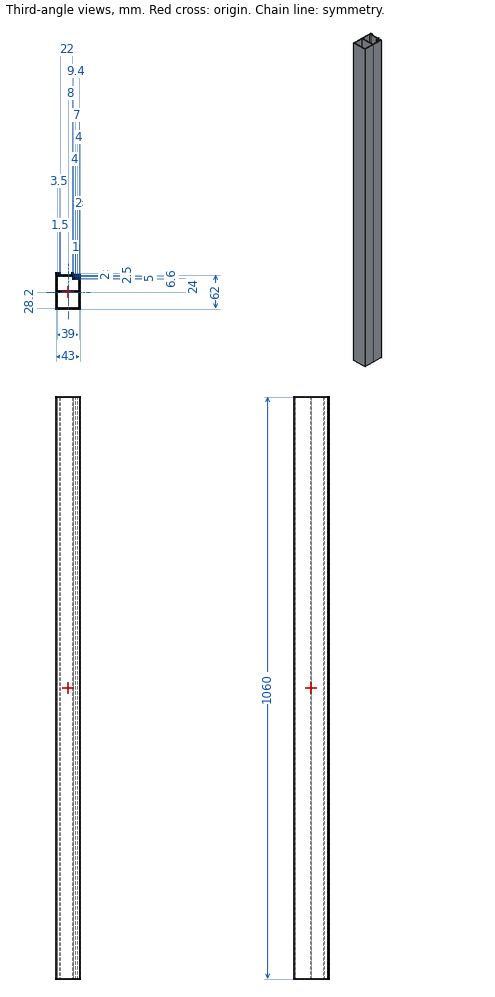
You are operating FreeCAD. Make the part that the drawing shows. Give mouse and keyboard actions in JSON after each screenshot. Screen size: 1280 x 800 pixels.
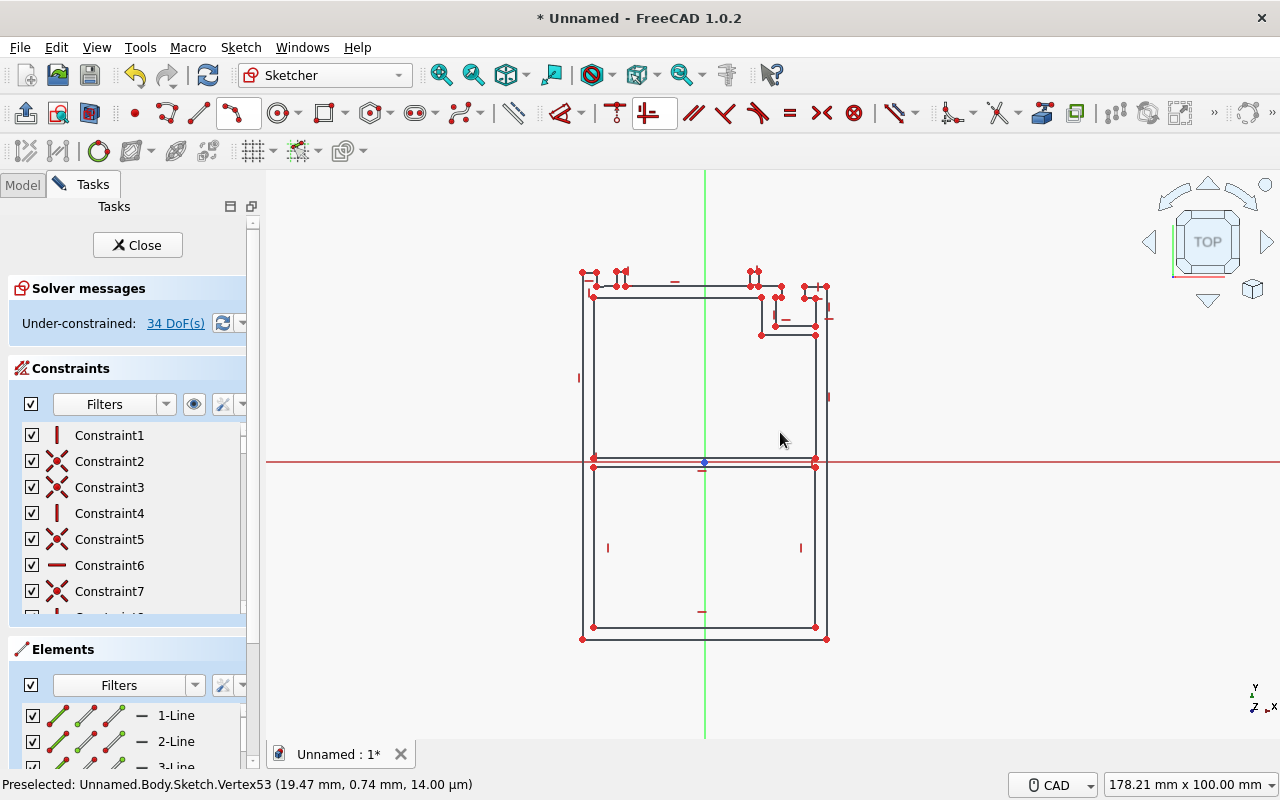
{"action": "scroll", "coordinate": [778, 298], "scroll_direction": "up", "scroll_amount": 9}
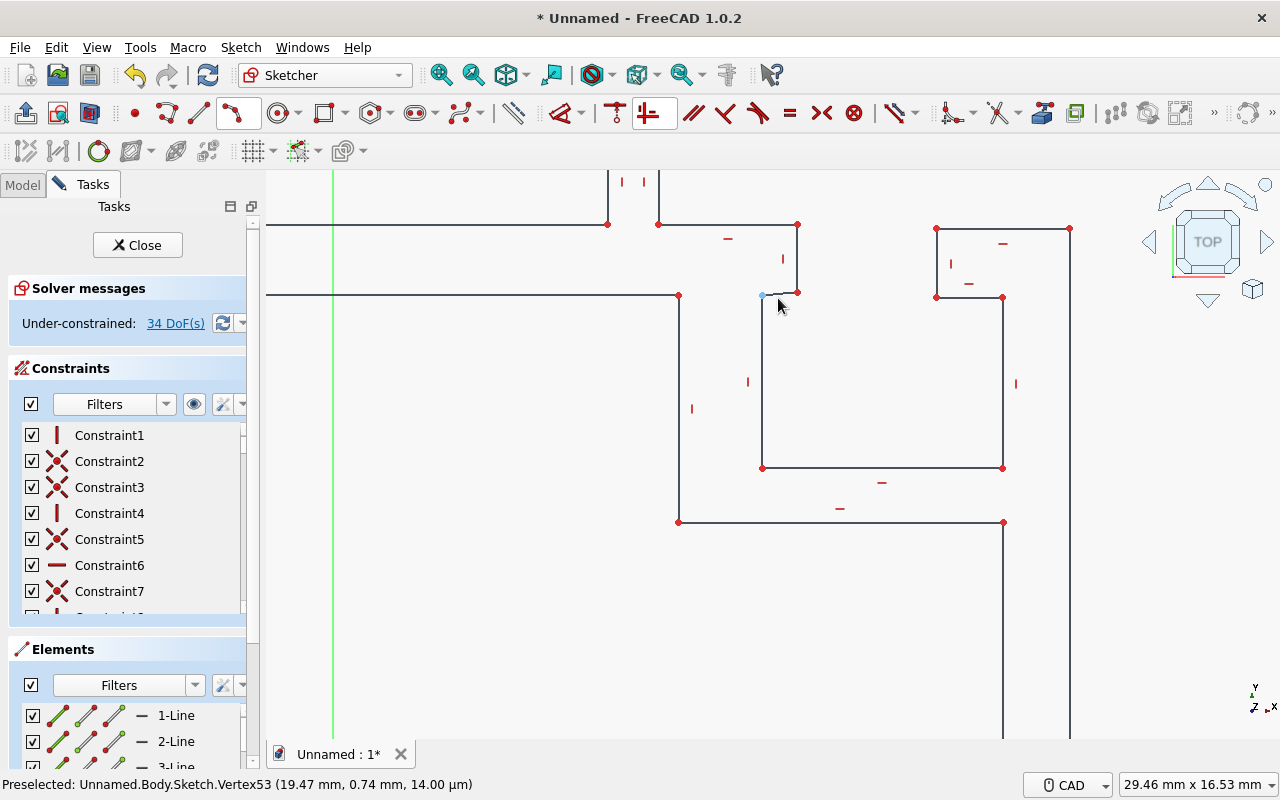
{"action": "left_click", "coordinate": [776, 294]}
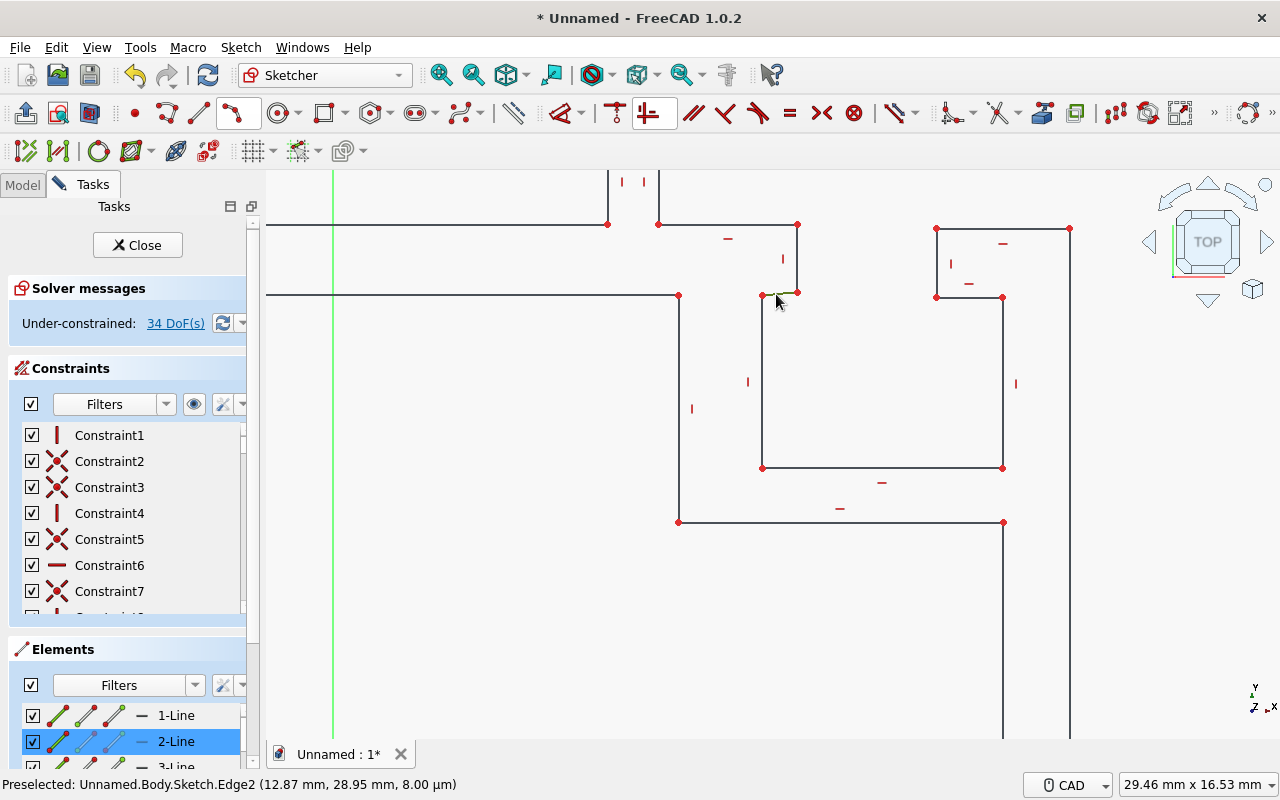
{"action": "left_click", "coordinate": [672, 114]}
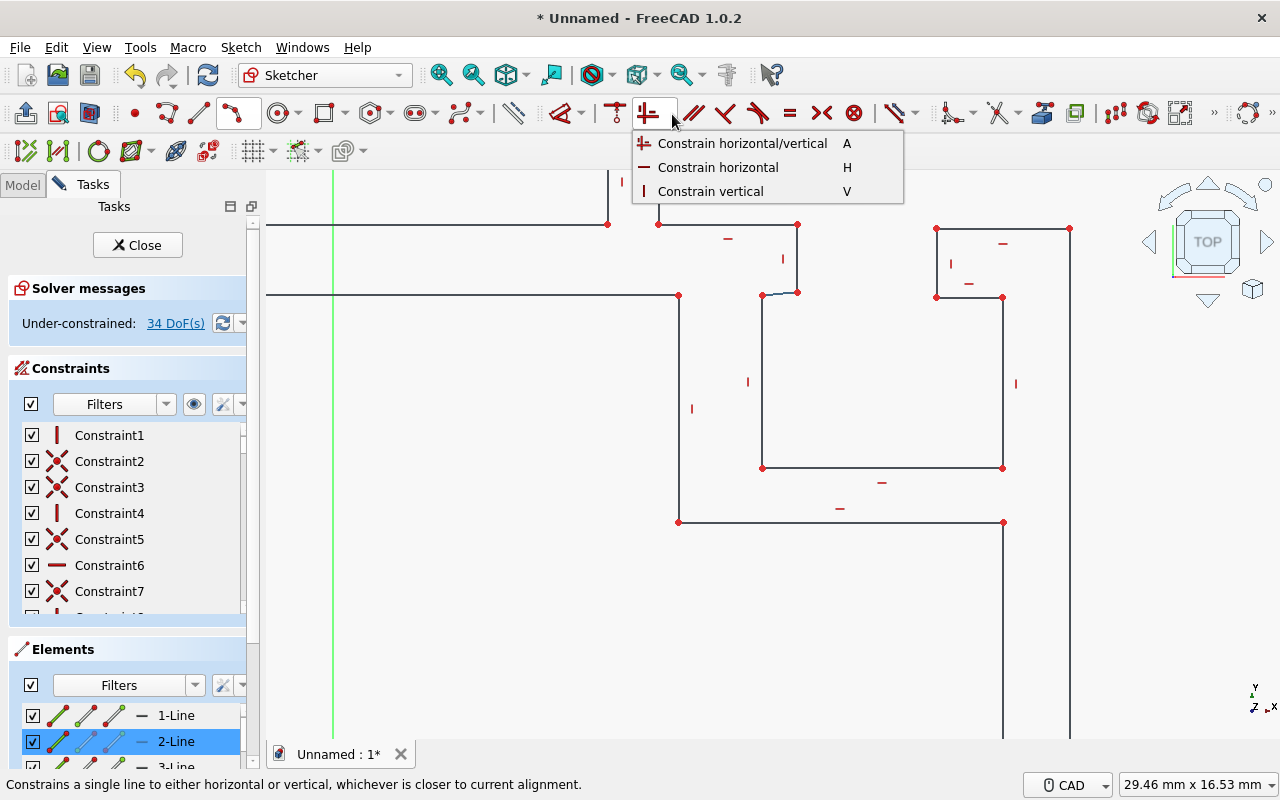
{"action": "left_click", "coordinate": [768, 167]}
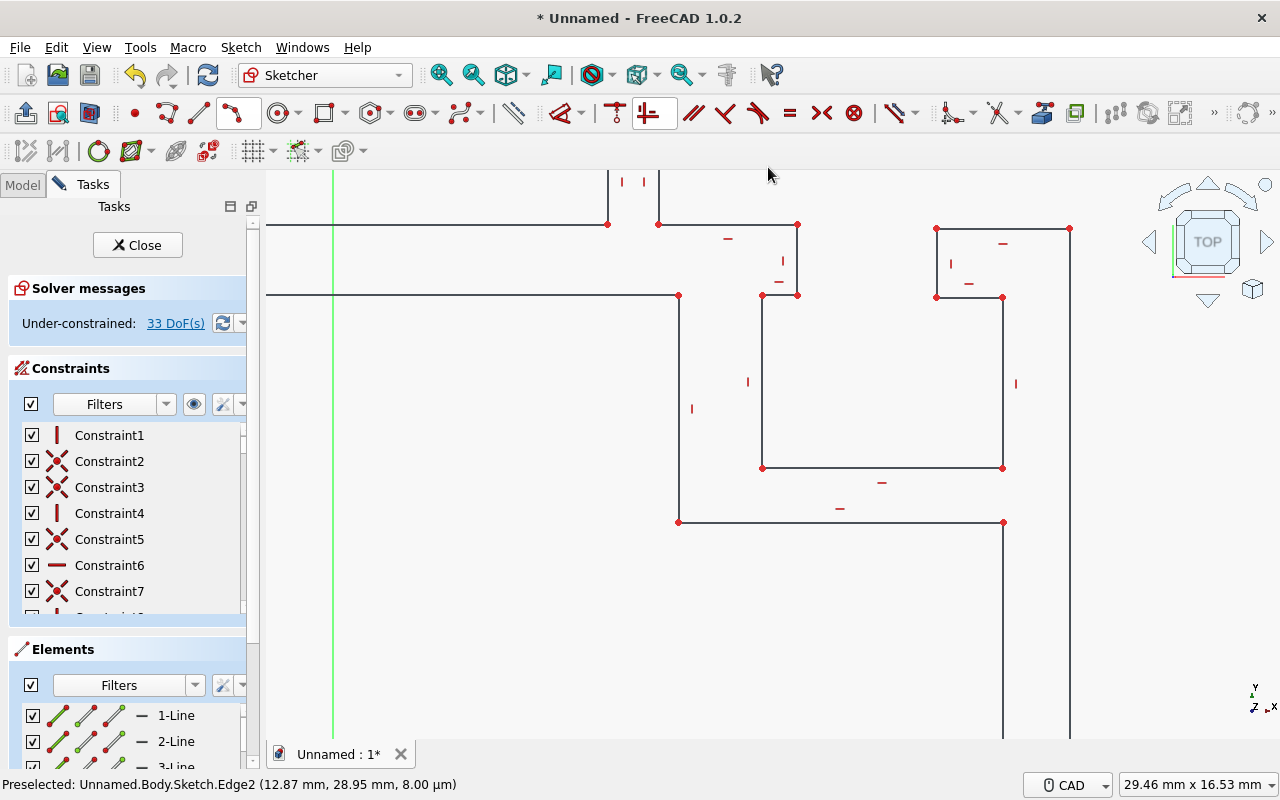
{"action": "scroll", "coordinate": [778, 297], "scroll_direction": "down", "scroll_amount": 9}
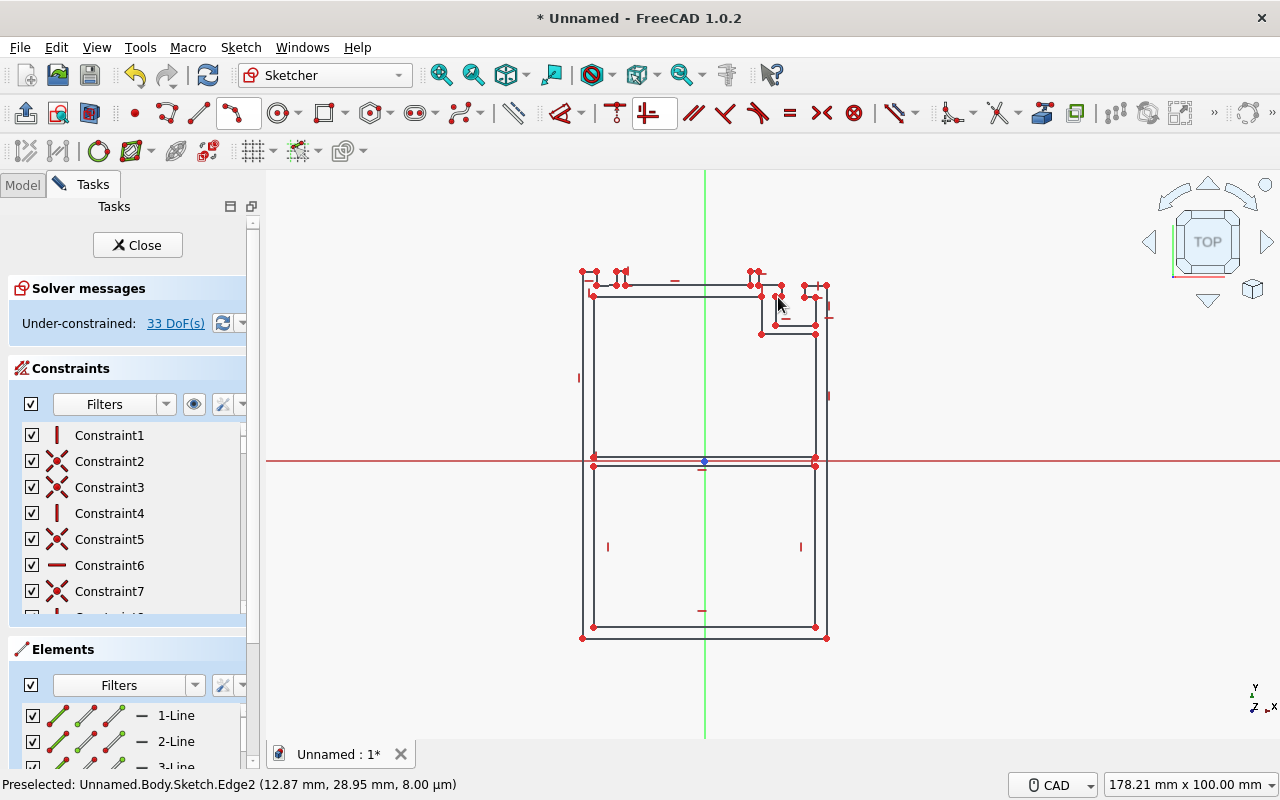
{"action": "scroll", "coordinate": [611, 285], "scroll_direction": "up", "scroll_amount": 5}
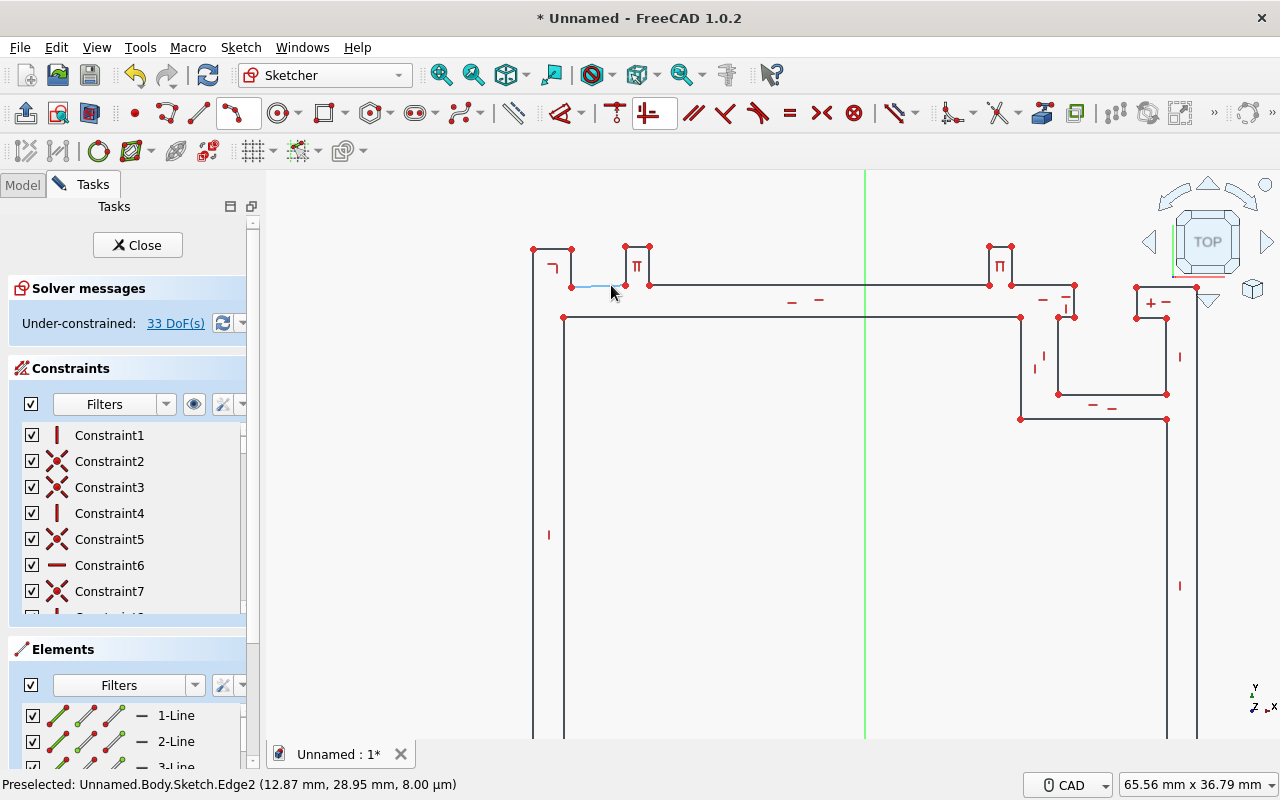
{"action": "left_click", "coordinate": [609, 286]}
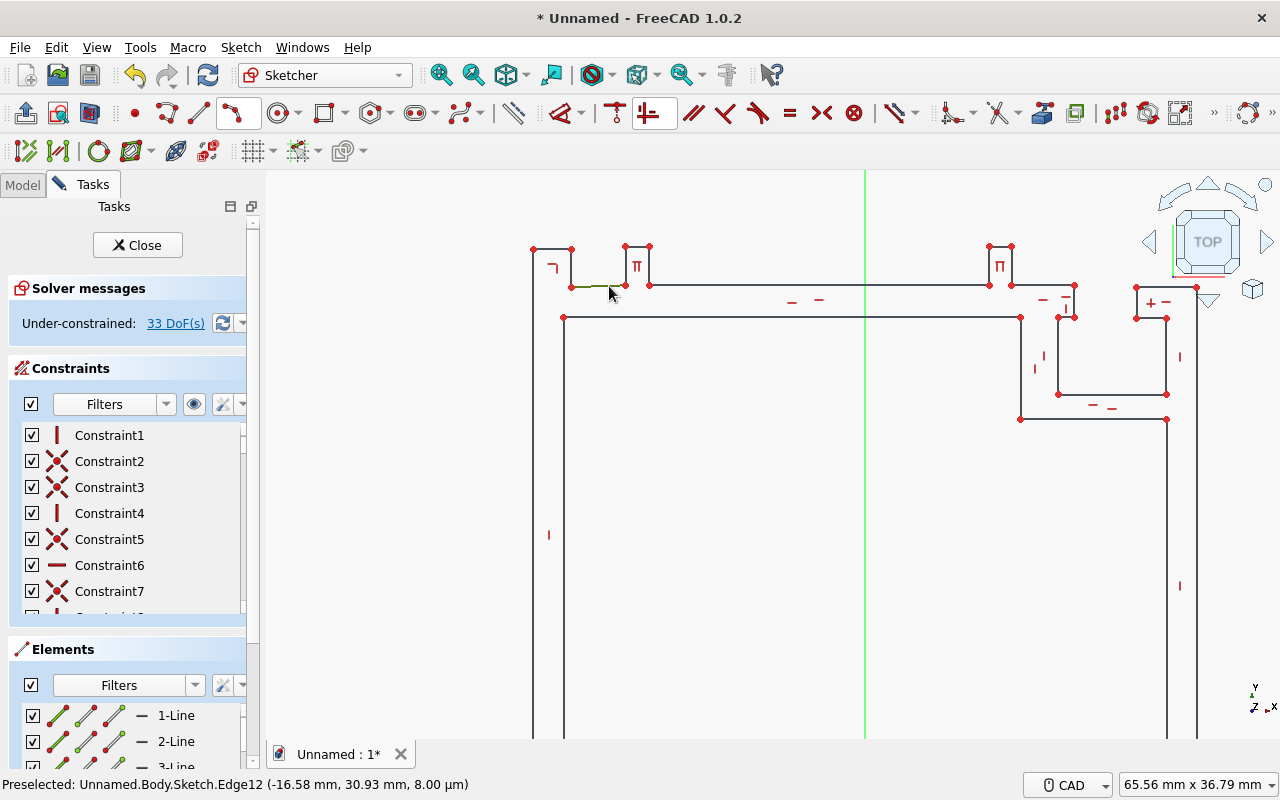
{"action": "left_click", "coordinate": [672, 114]}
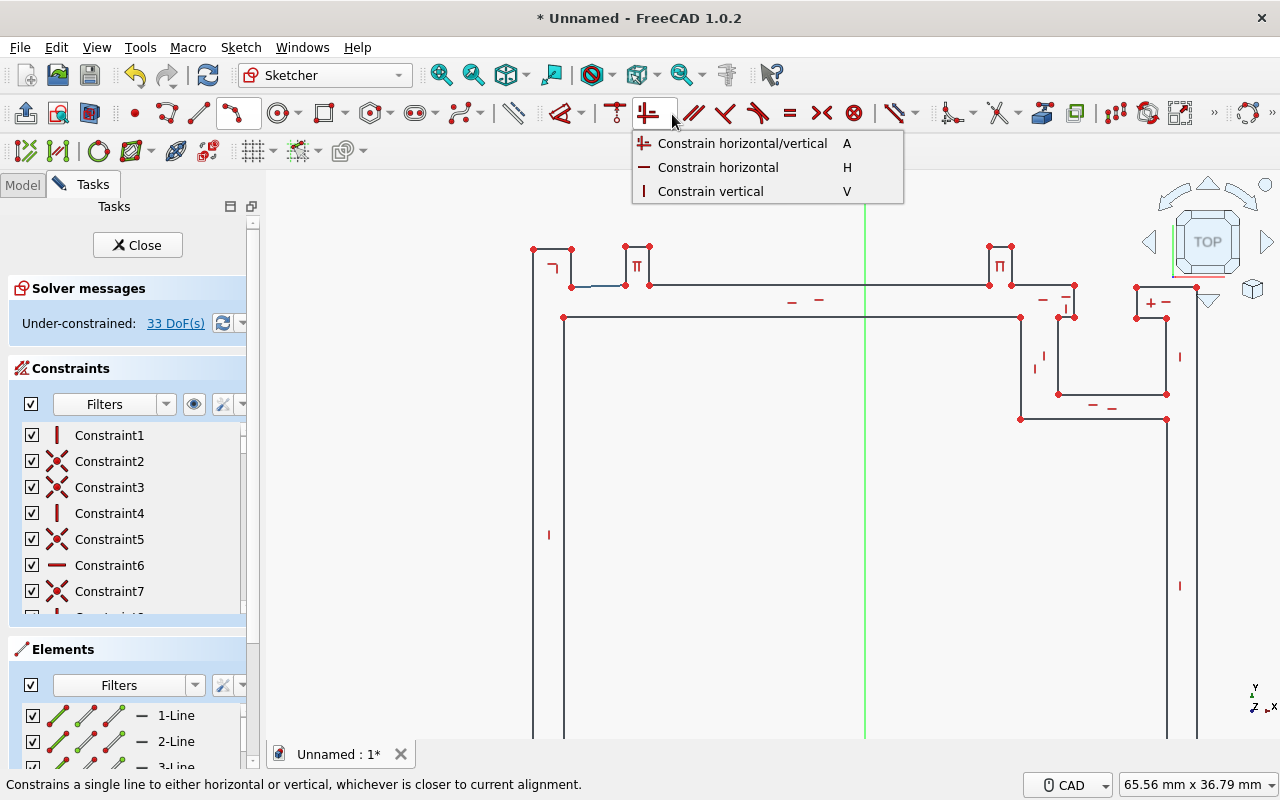
{"action": "left_click", "coordinate": [768, 167]}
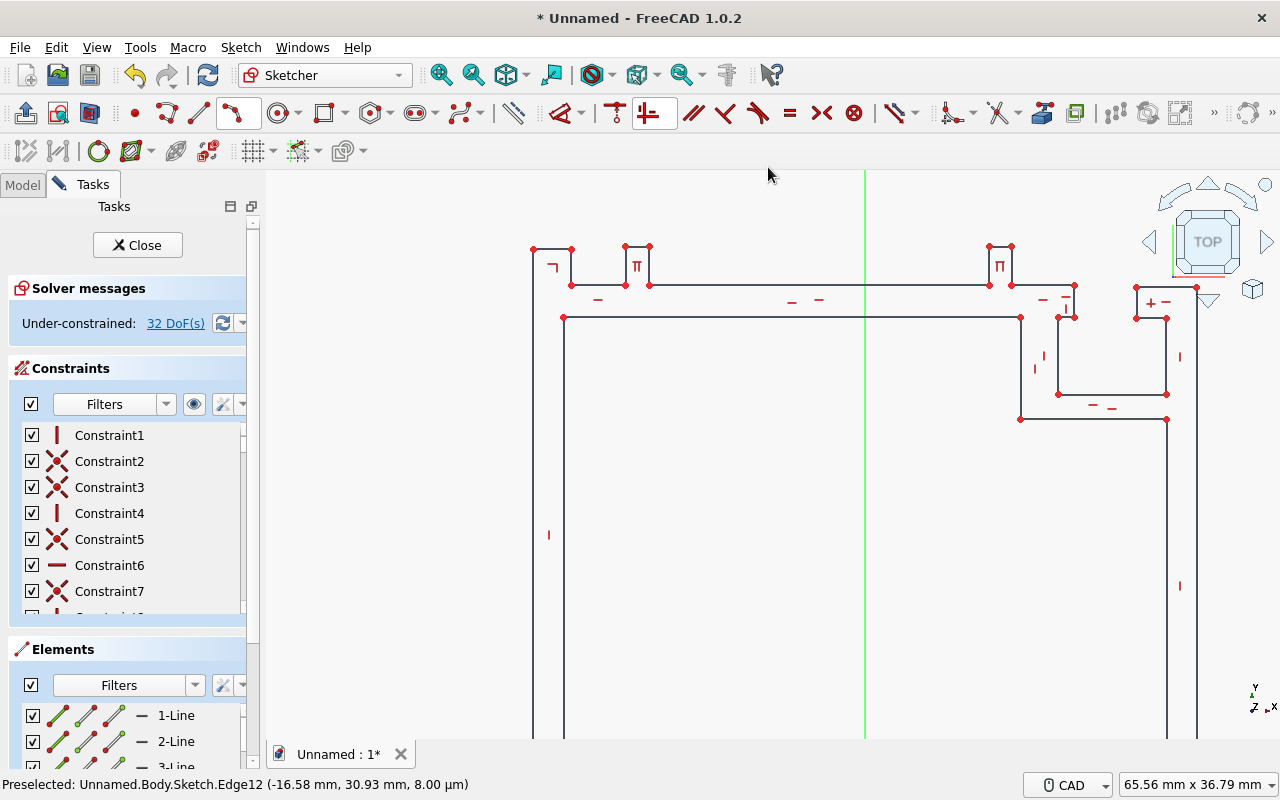
{"action": "scroll", "coordinate": [611, 285], "scroll_direction": "down", "scroll_amount": 5}